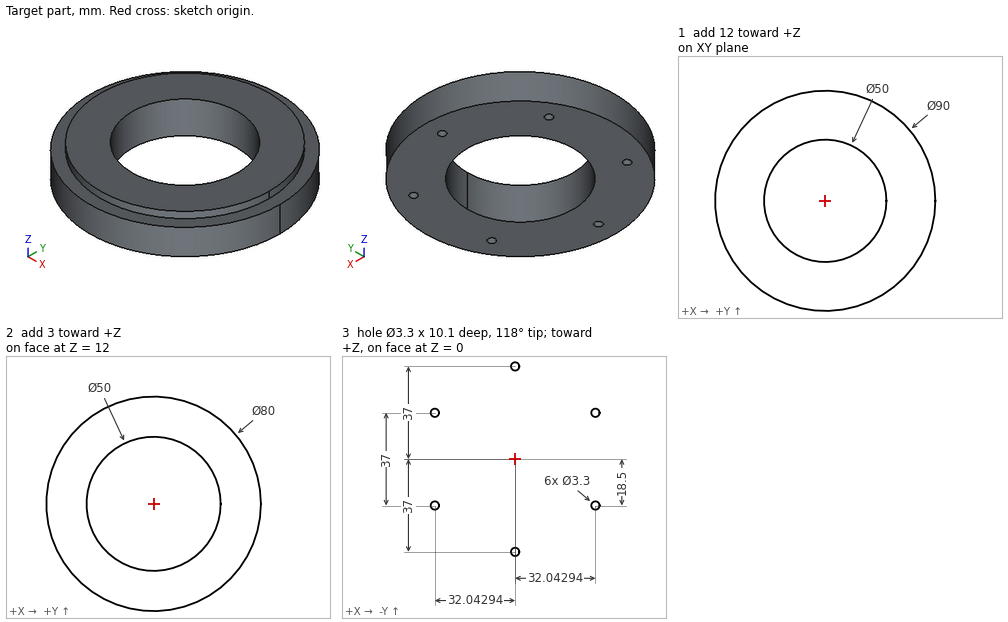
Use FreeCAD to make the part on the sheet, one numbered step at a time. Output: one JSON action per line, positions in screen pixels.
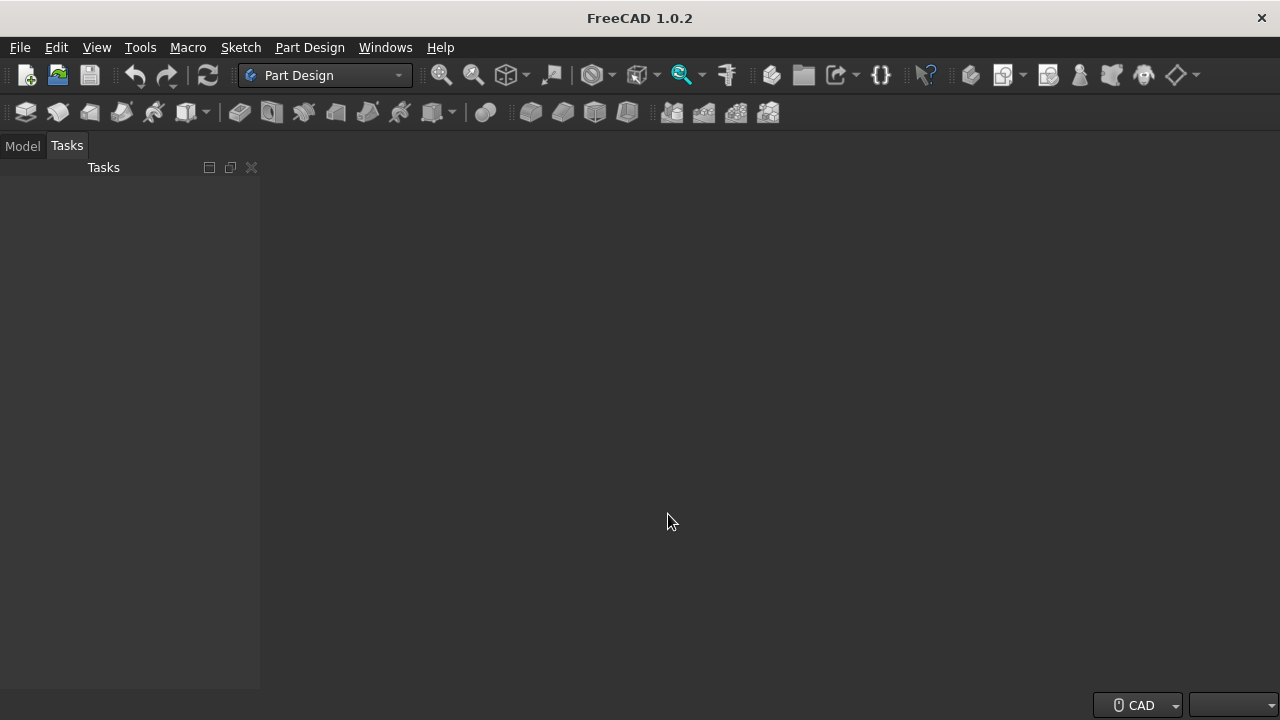
{"action": "left_click", "coordinate": [26, 76]}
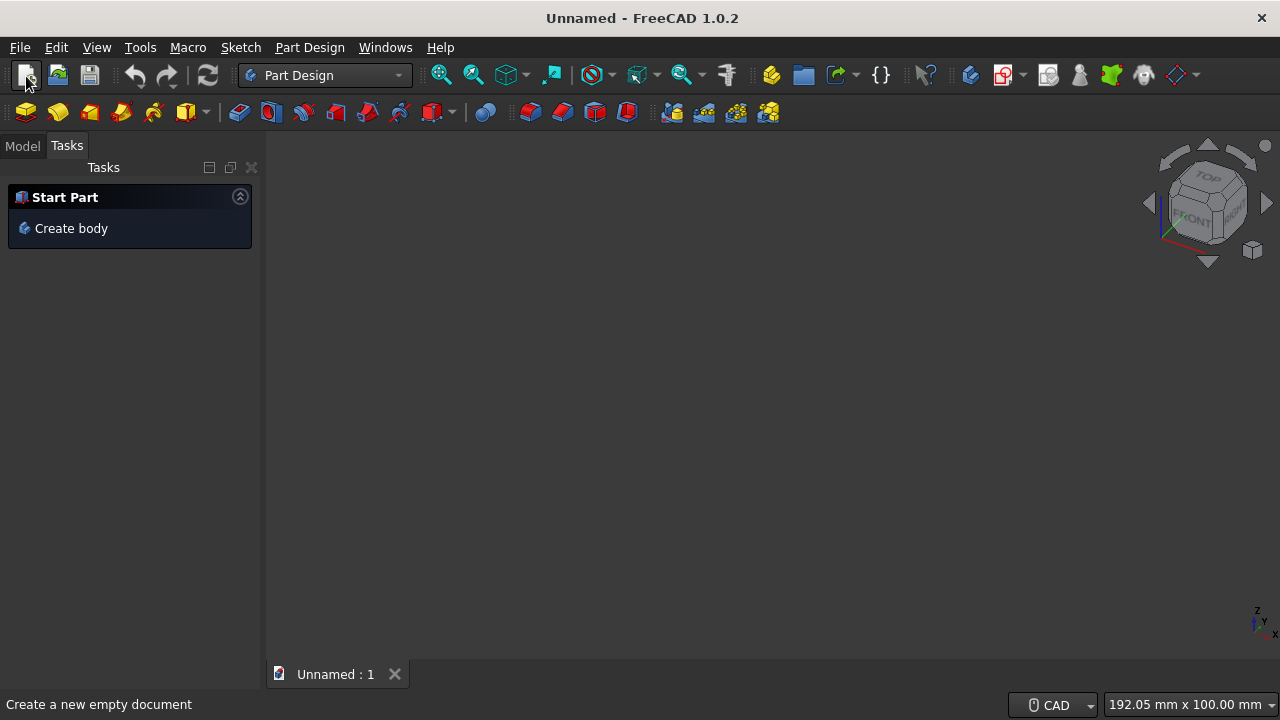
{"action": "left_click", "coordinate": [1004, 76]}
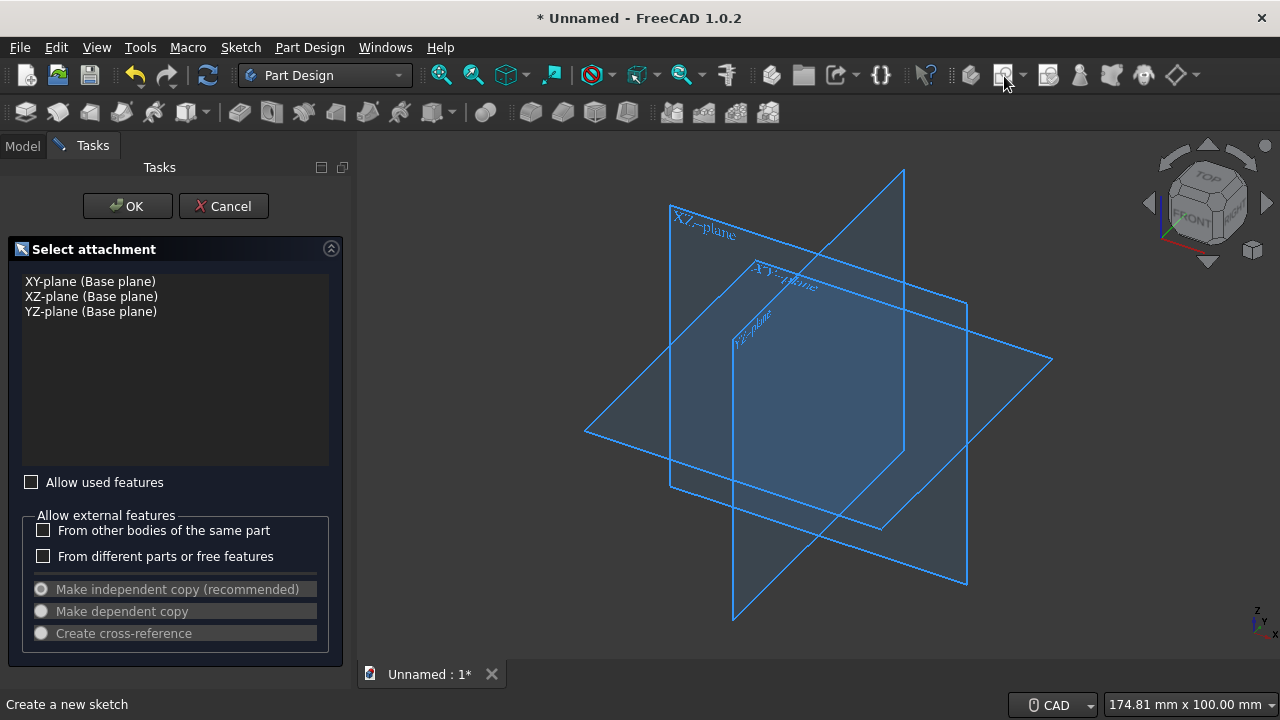
{"action": "left_click", "coordinate": [82, 282]}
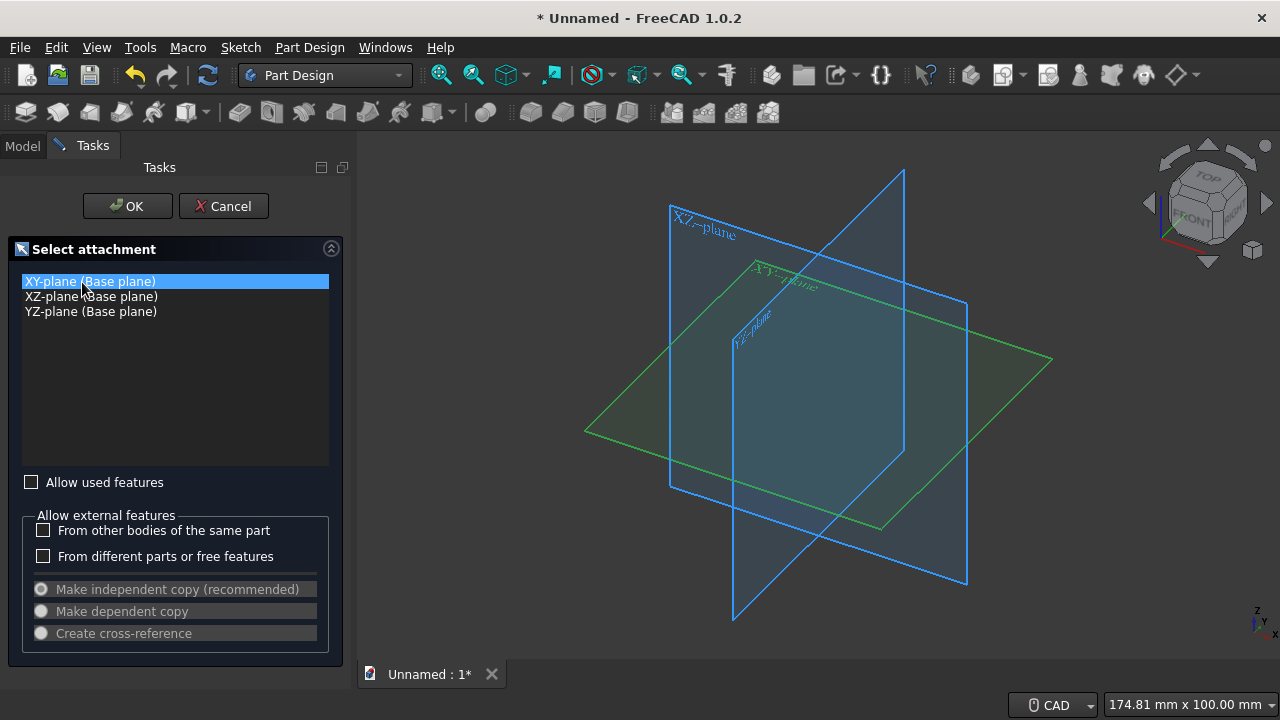
{"action": "left_click", "coordinate": [128, 206]}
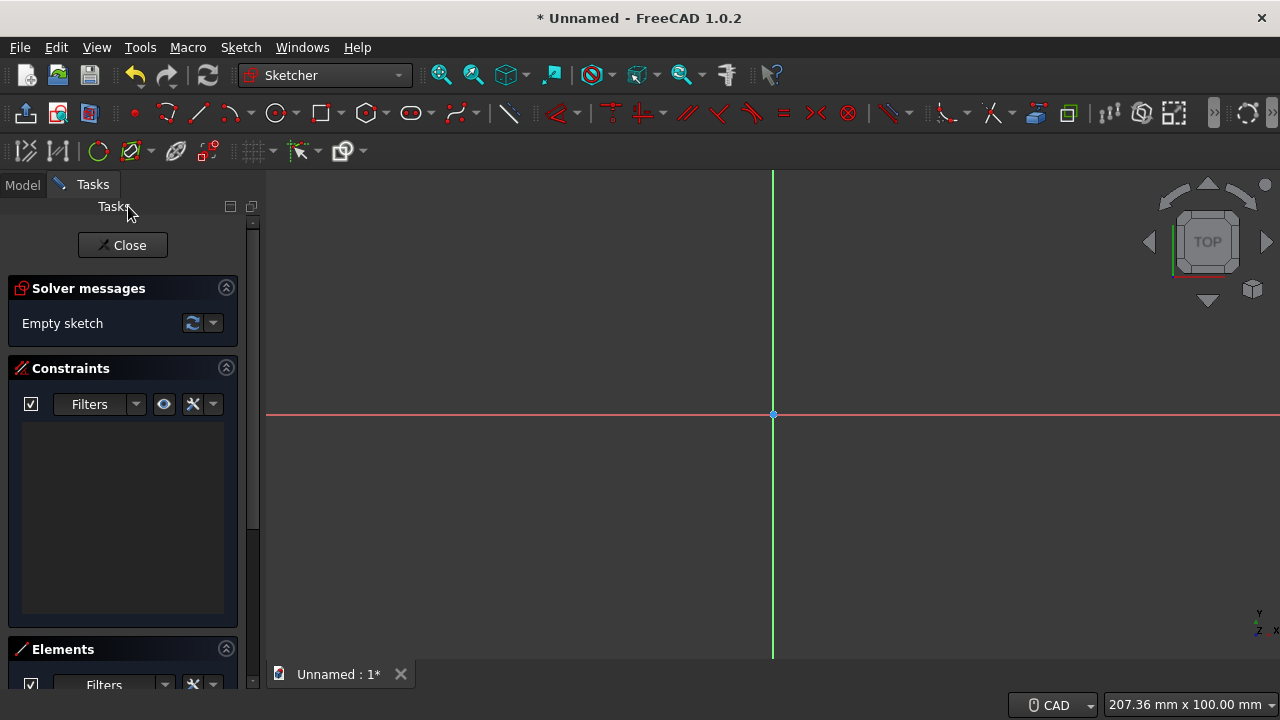
{"action": "scroll", "coordinate": [565, 414], "scroll_direction": "down", "scroll_amount": 2}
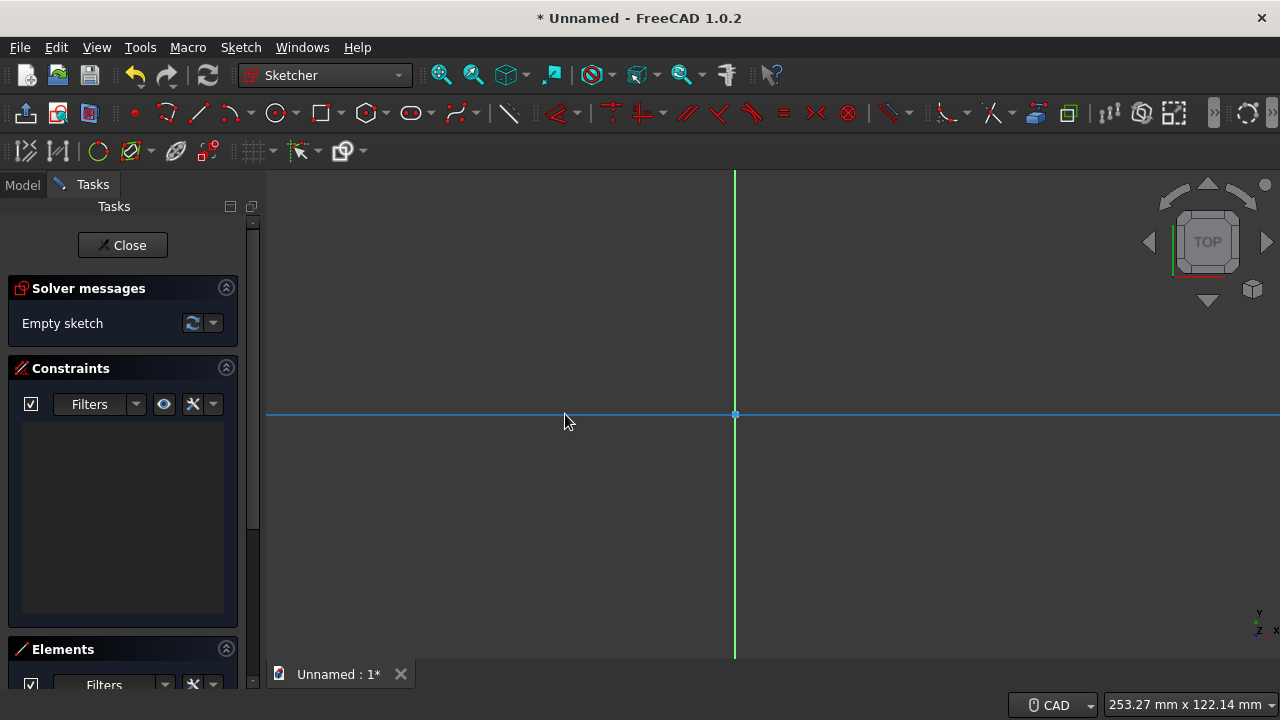
{"action": "left_click", "coordinate": [276, 114]}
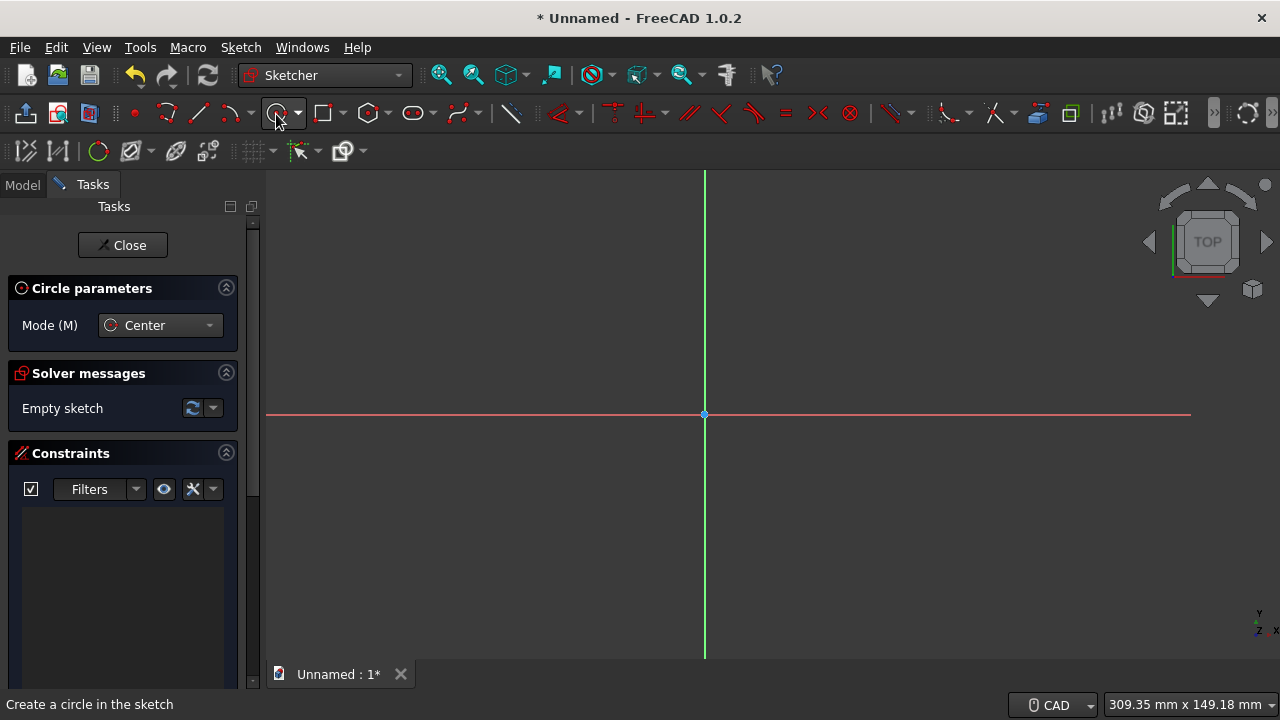
{"action": "left_click", "coordinate": [705, 414]}
{"action": "left_click", "coordinate": [809, 310]}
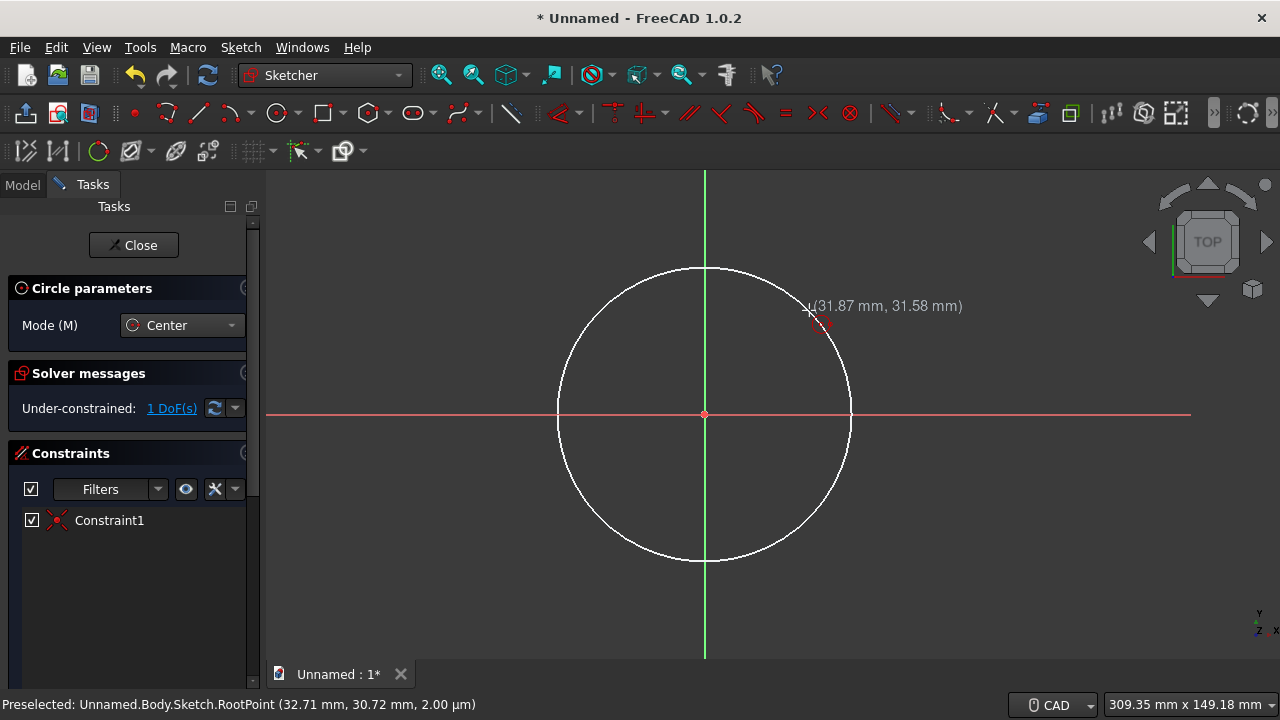
{"action": "left_click", "coordinate": [705, 414]}
{"action": "left_click", "coordinate": [762, 357]}
{"action": "key", "text": "Escape"}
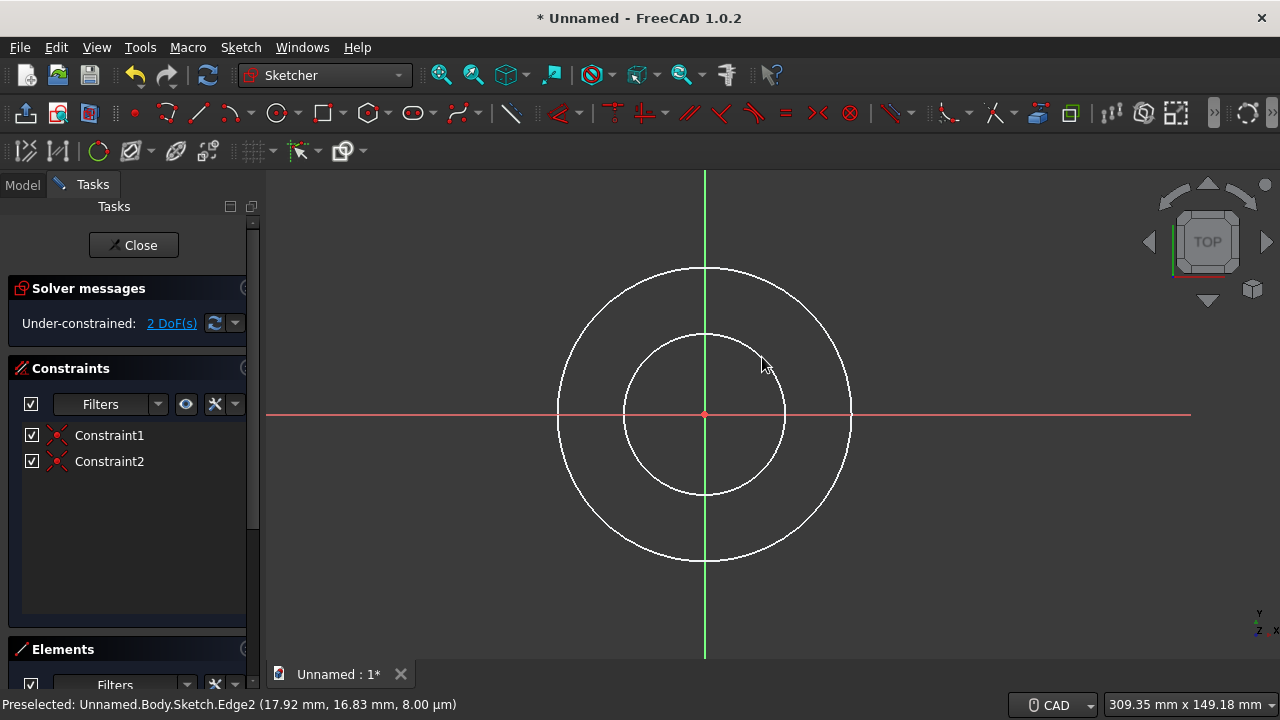
{"action": "left_click", "coordinate": [558, 114]}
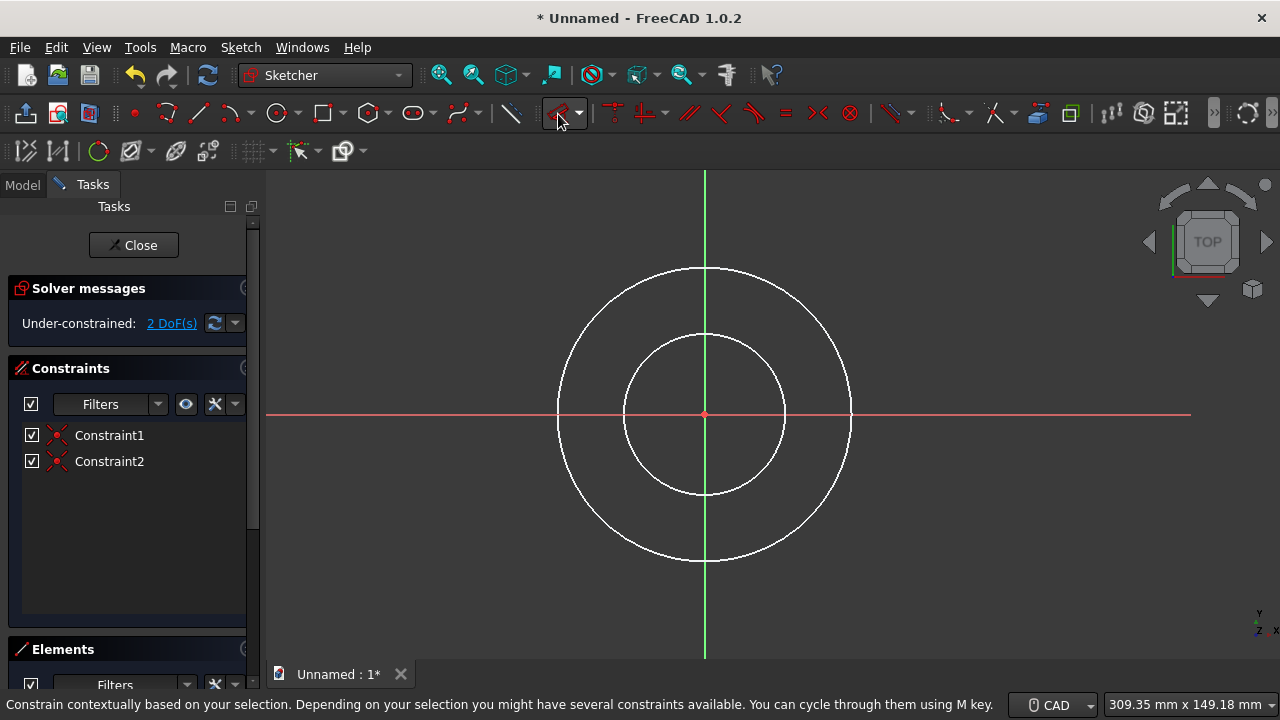
{"action": "left_click", "coordinate": [808, 310]}
{"action": "left_click", "coordinate": [831, 287]}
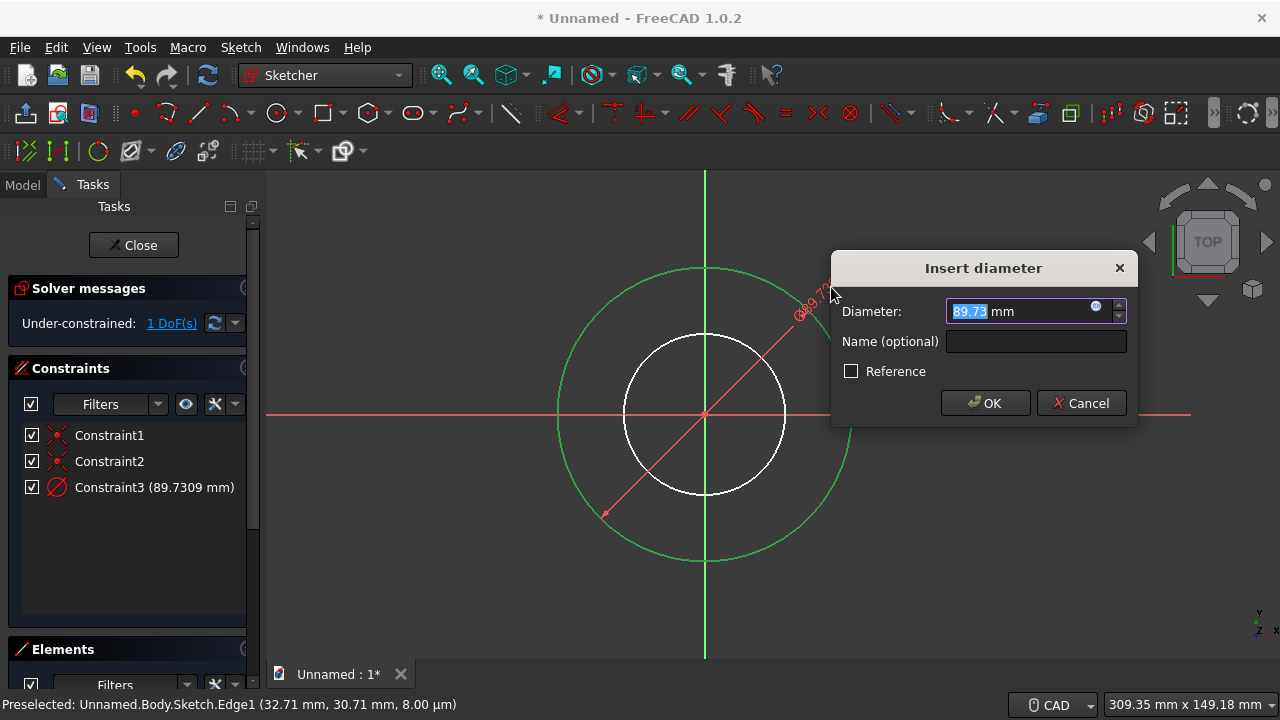
{"action": "type", "text": "90"}
{"action": "key", "text": "Return"}